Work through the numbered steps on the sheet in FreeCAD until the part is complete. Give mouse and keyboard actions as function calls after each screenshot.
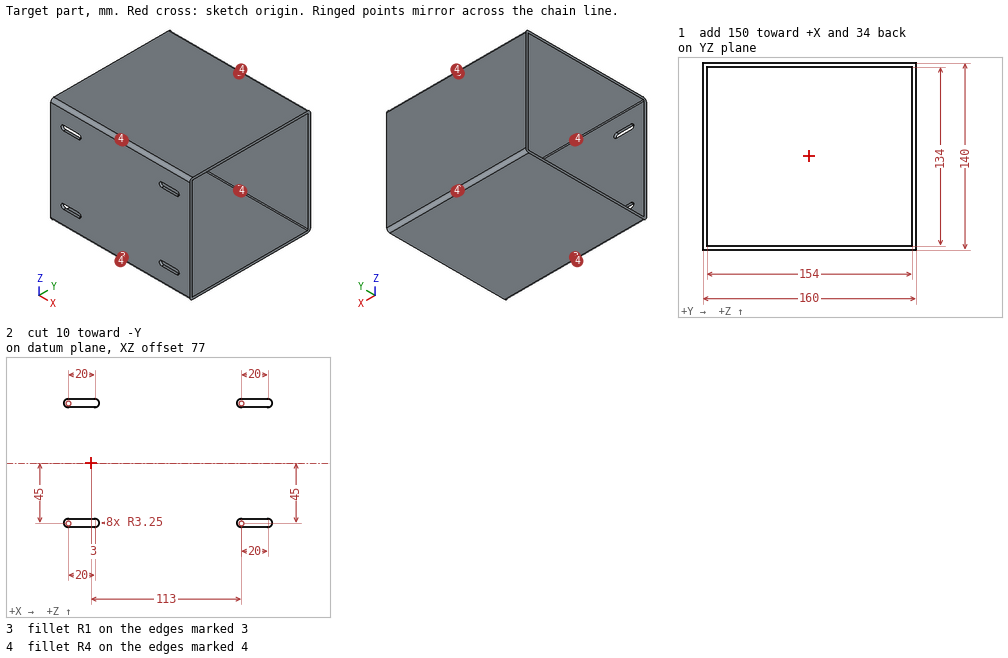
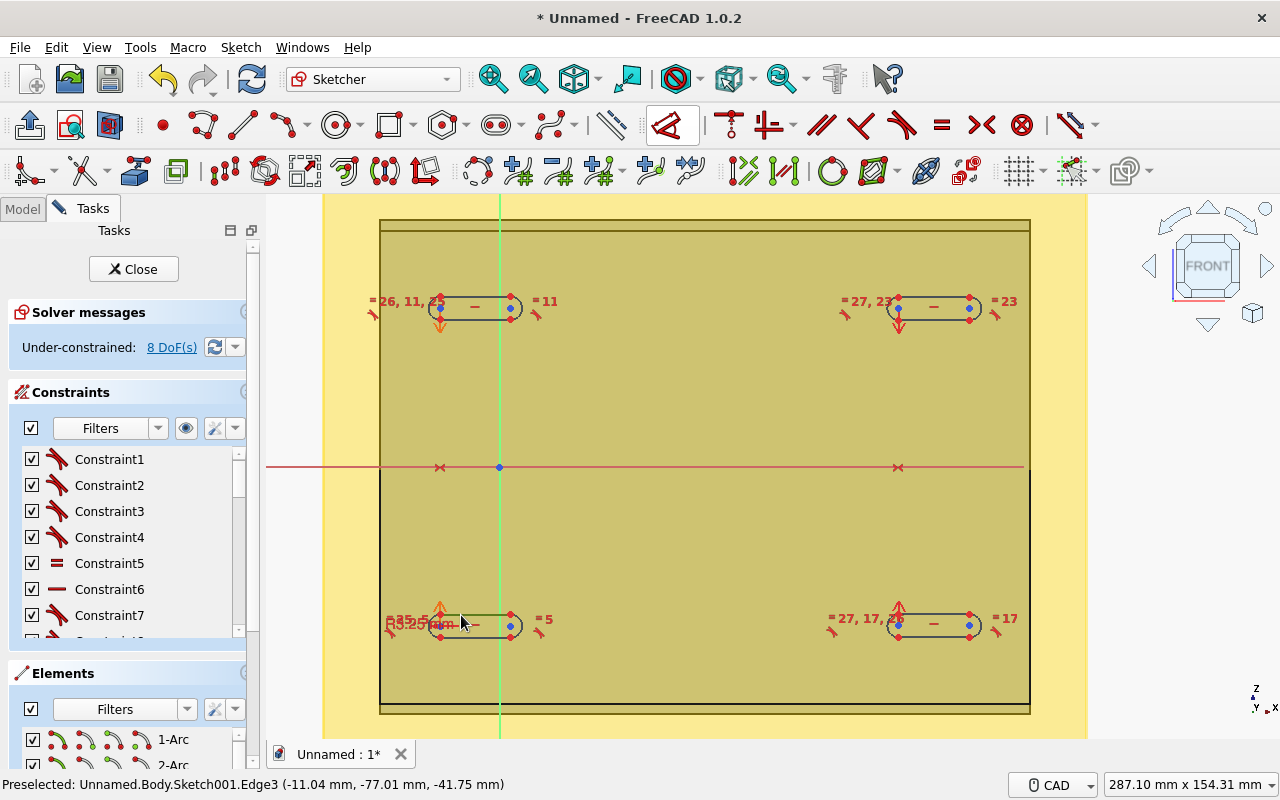
key(l)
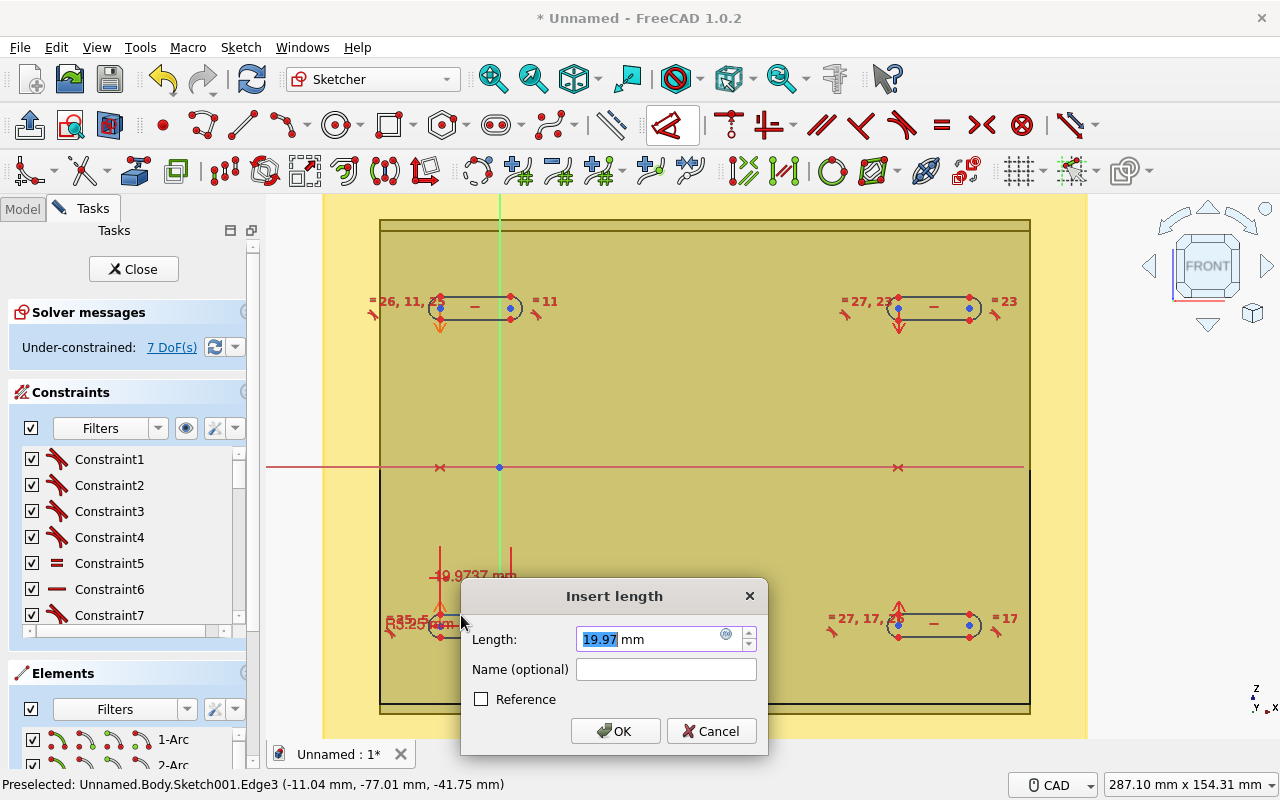
text(20)
key(Return)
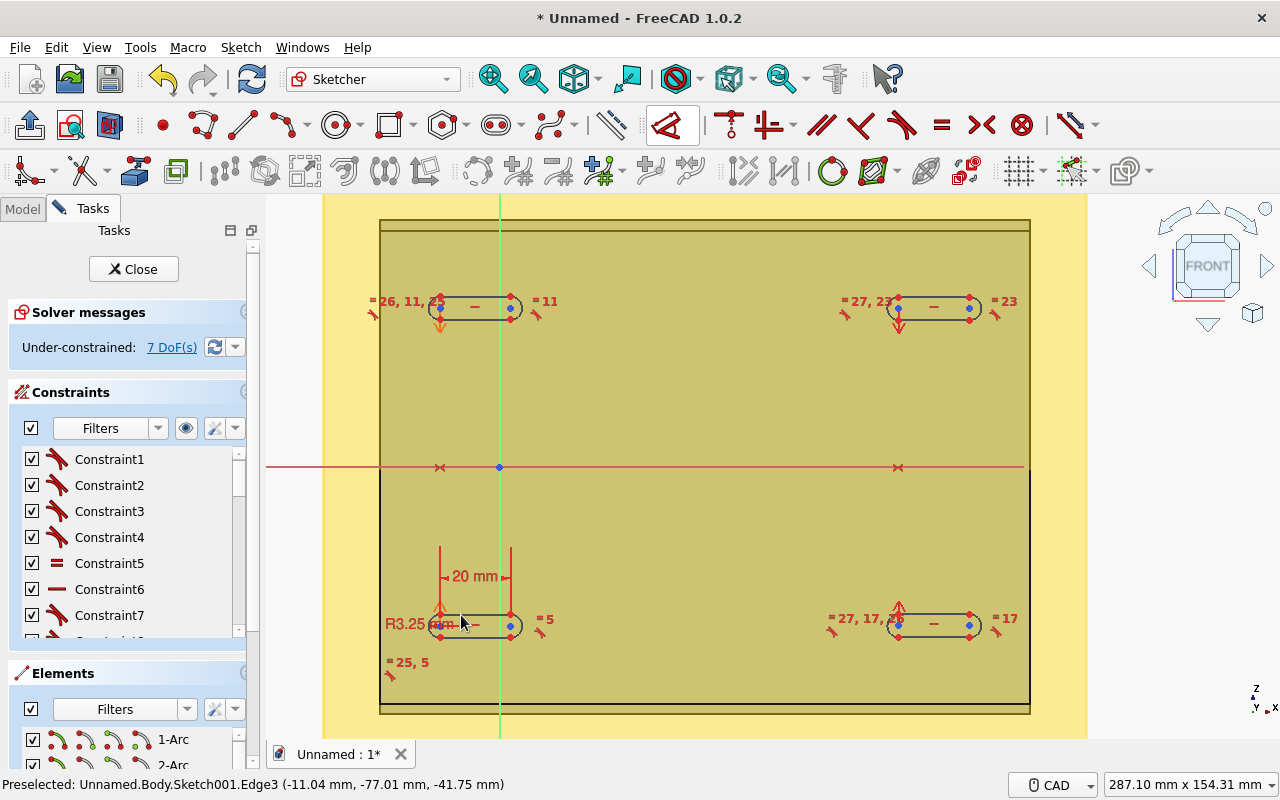
click(461, 297)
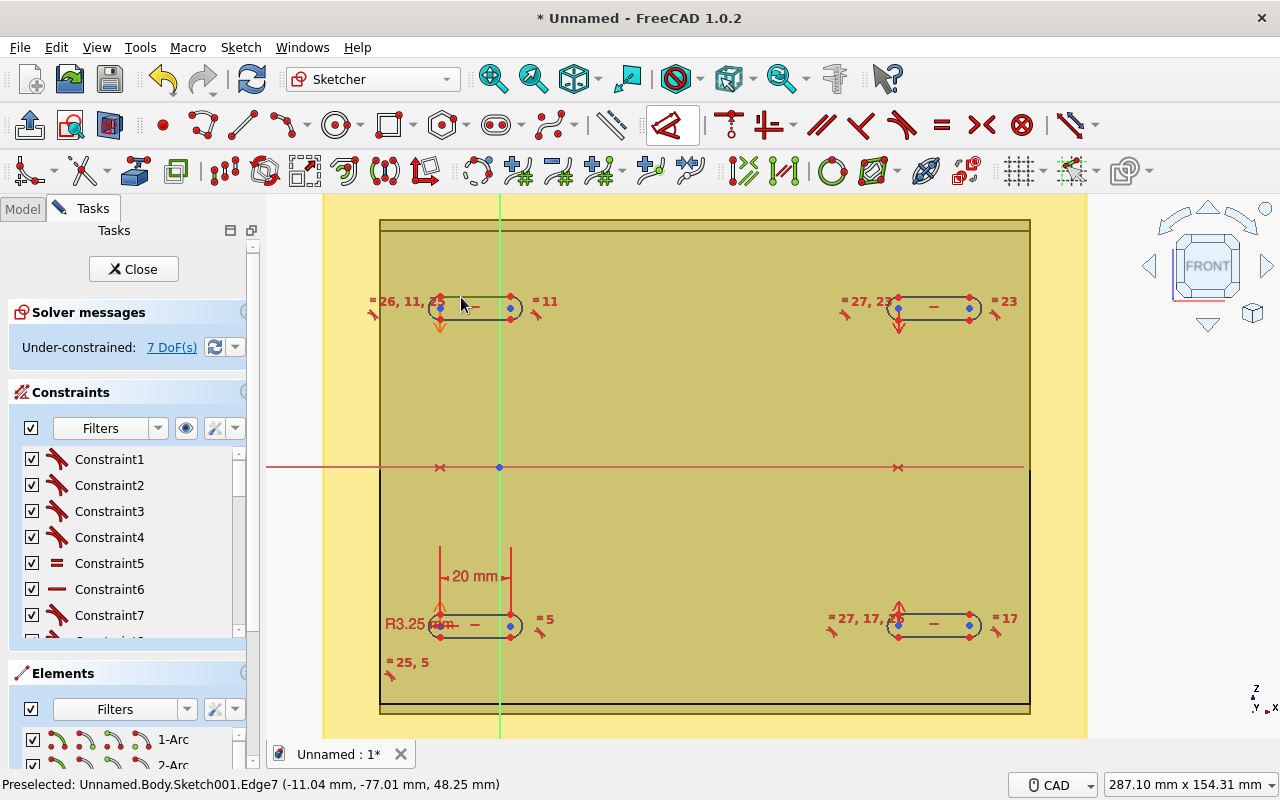
key(l)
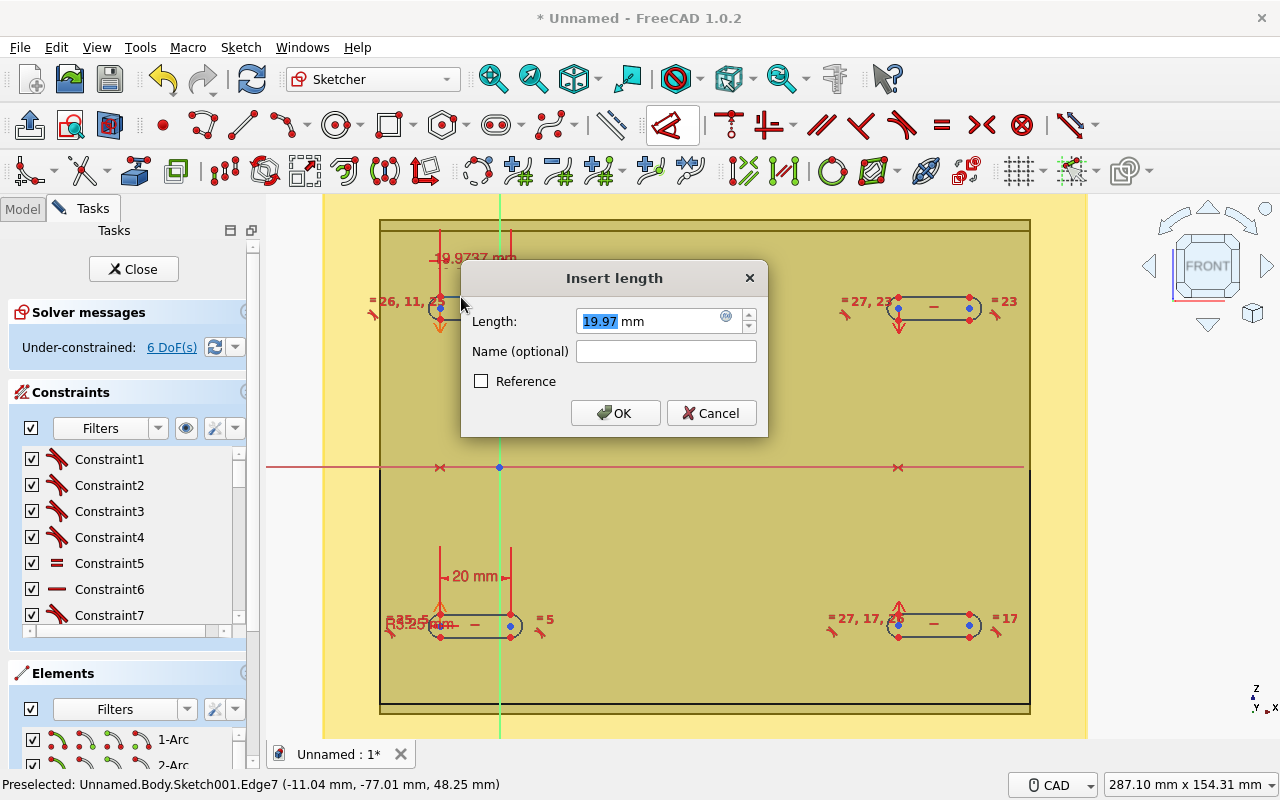
text(20)
key(Return)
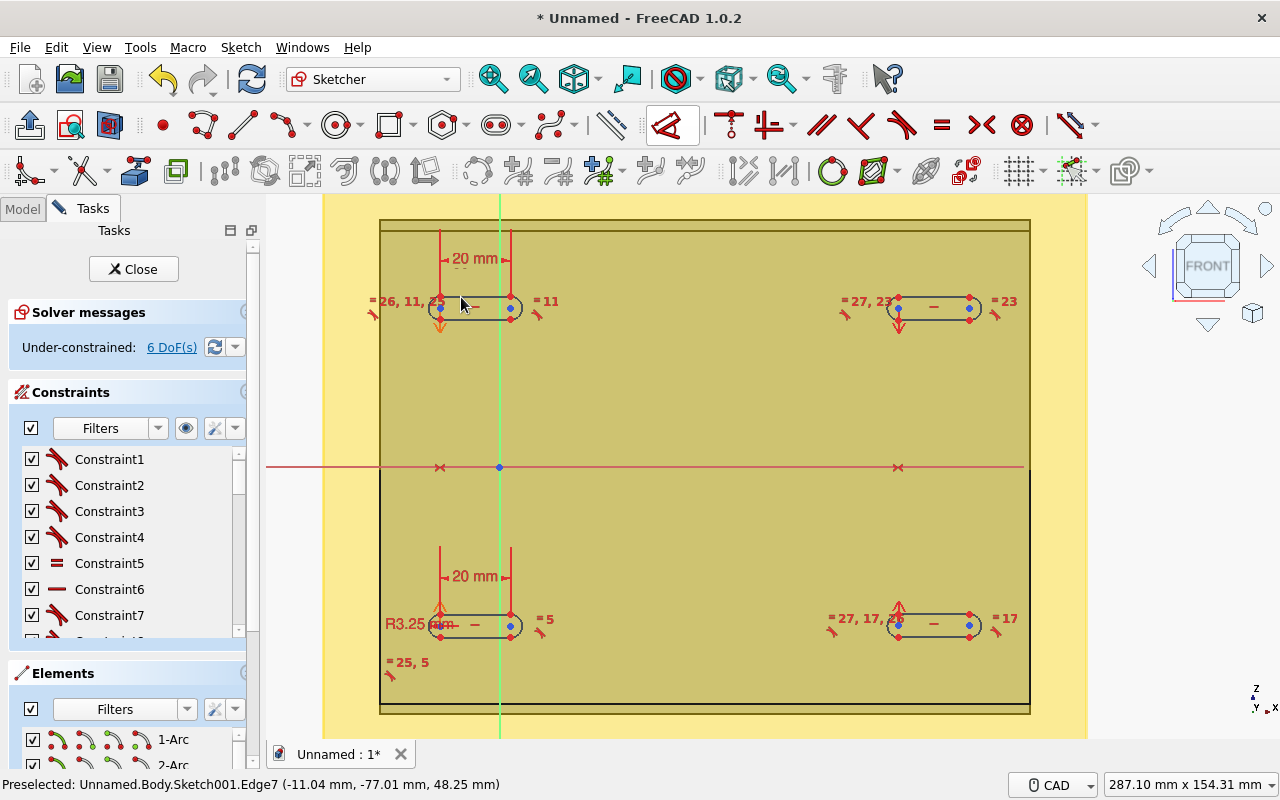
click(920, 614)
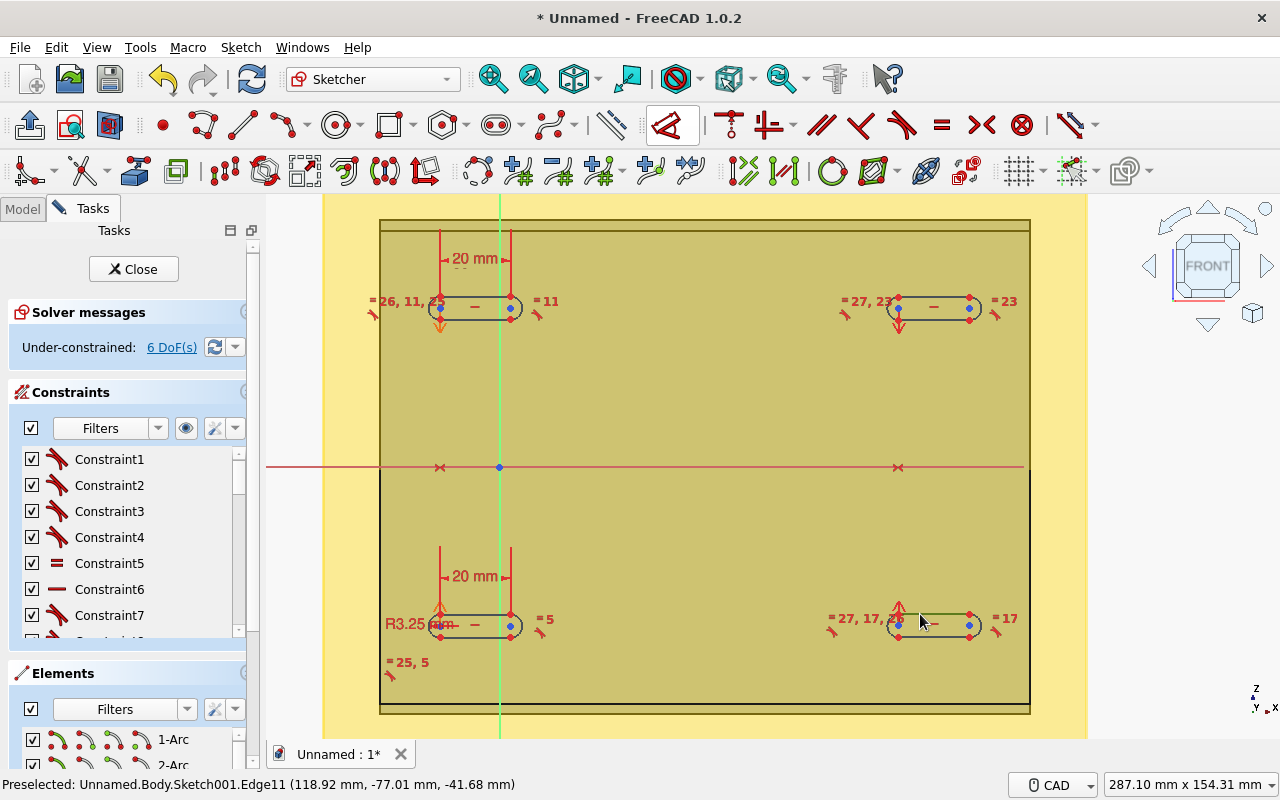
key(l)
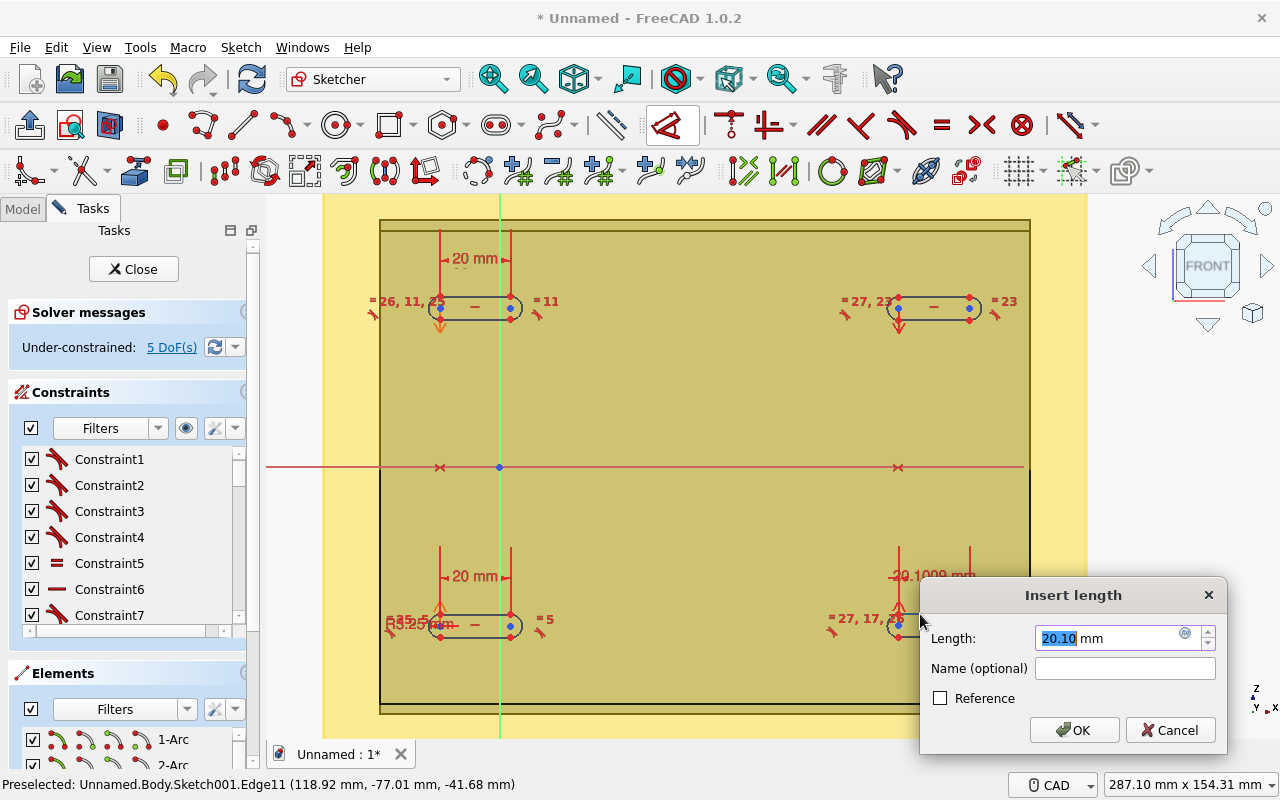
text(20)
key(Return)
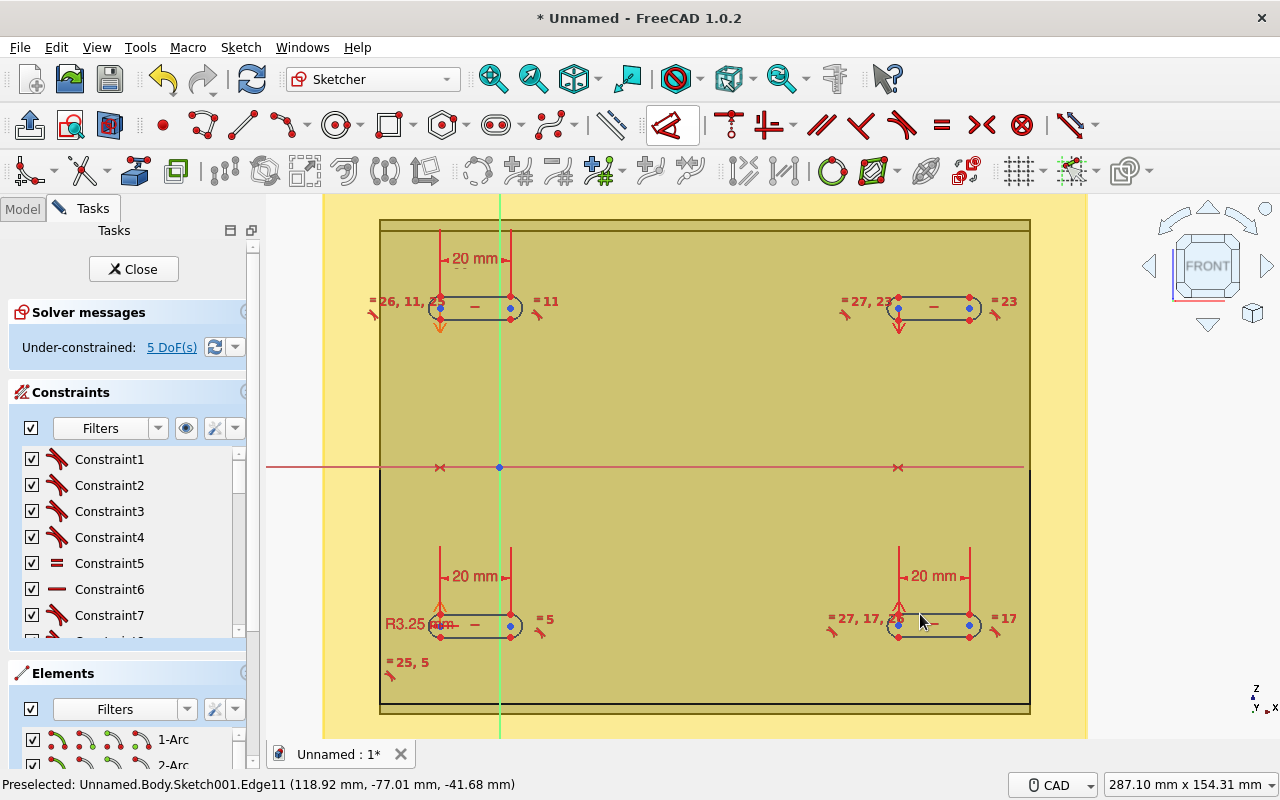
click(920, 297)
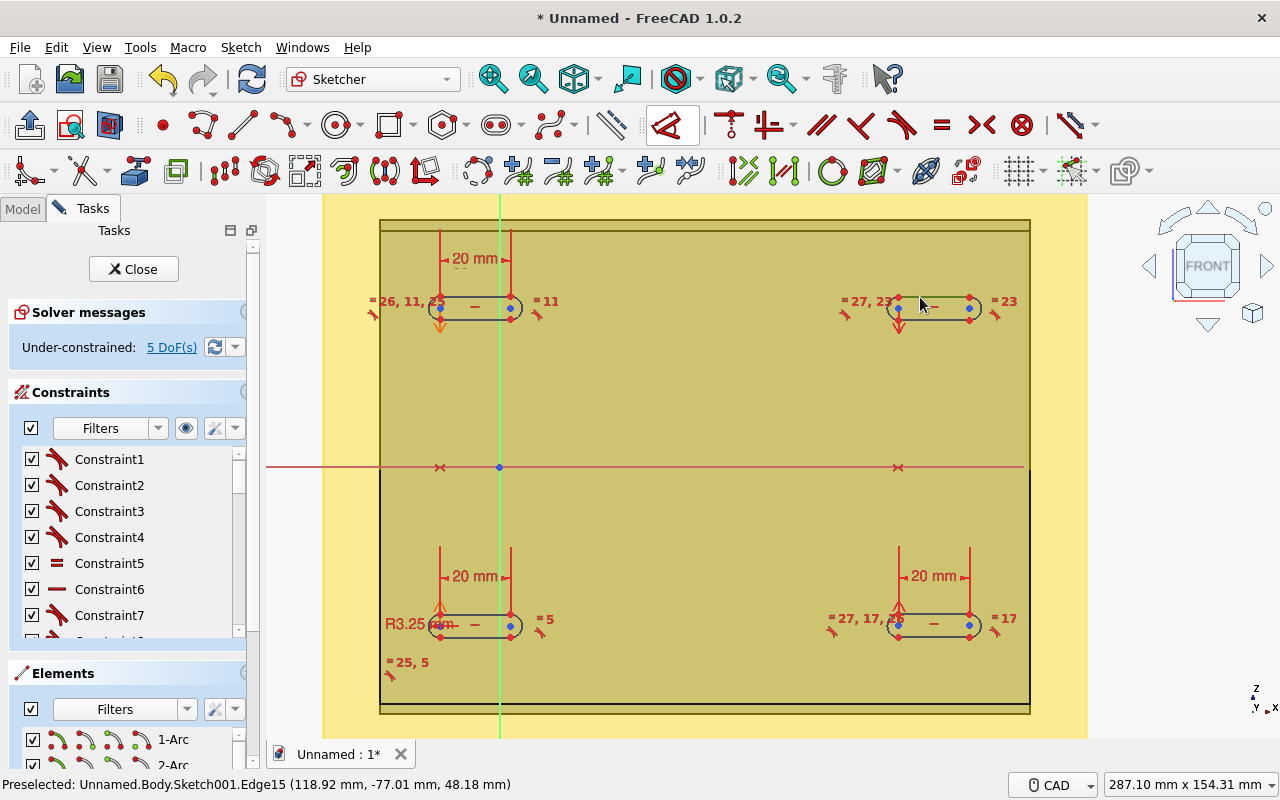
key(l)